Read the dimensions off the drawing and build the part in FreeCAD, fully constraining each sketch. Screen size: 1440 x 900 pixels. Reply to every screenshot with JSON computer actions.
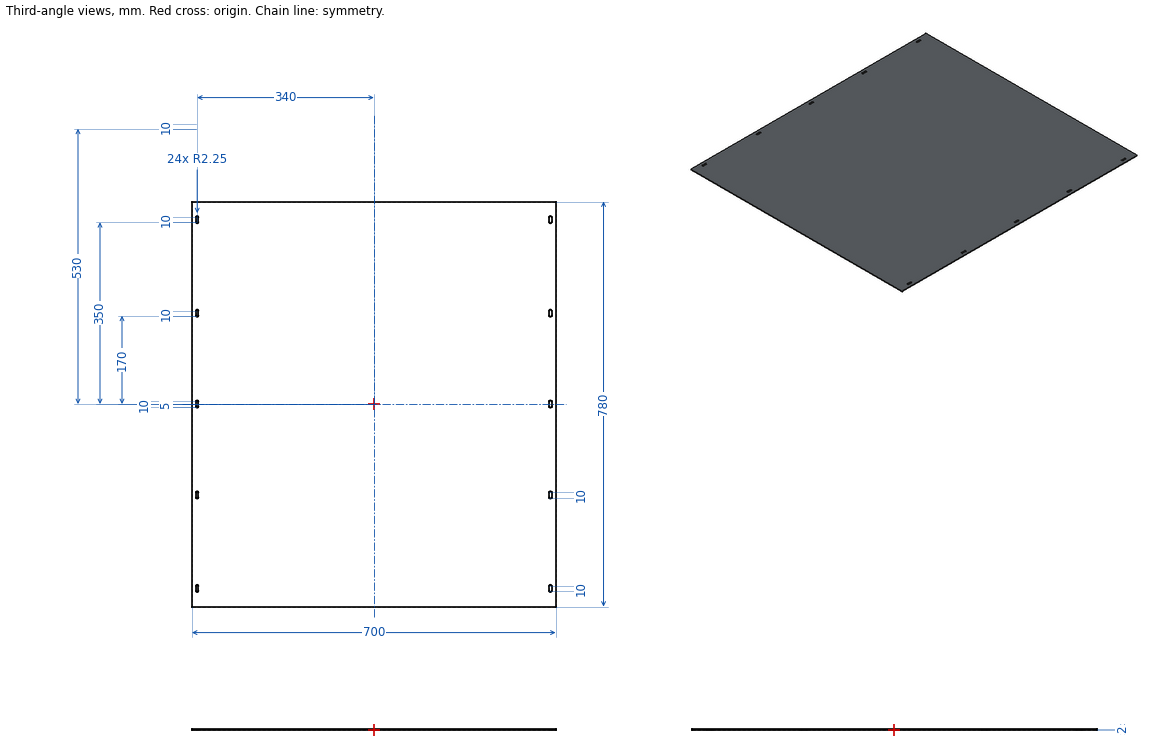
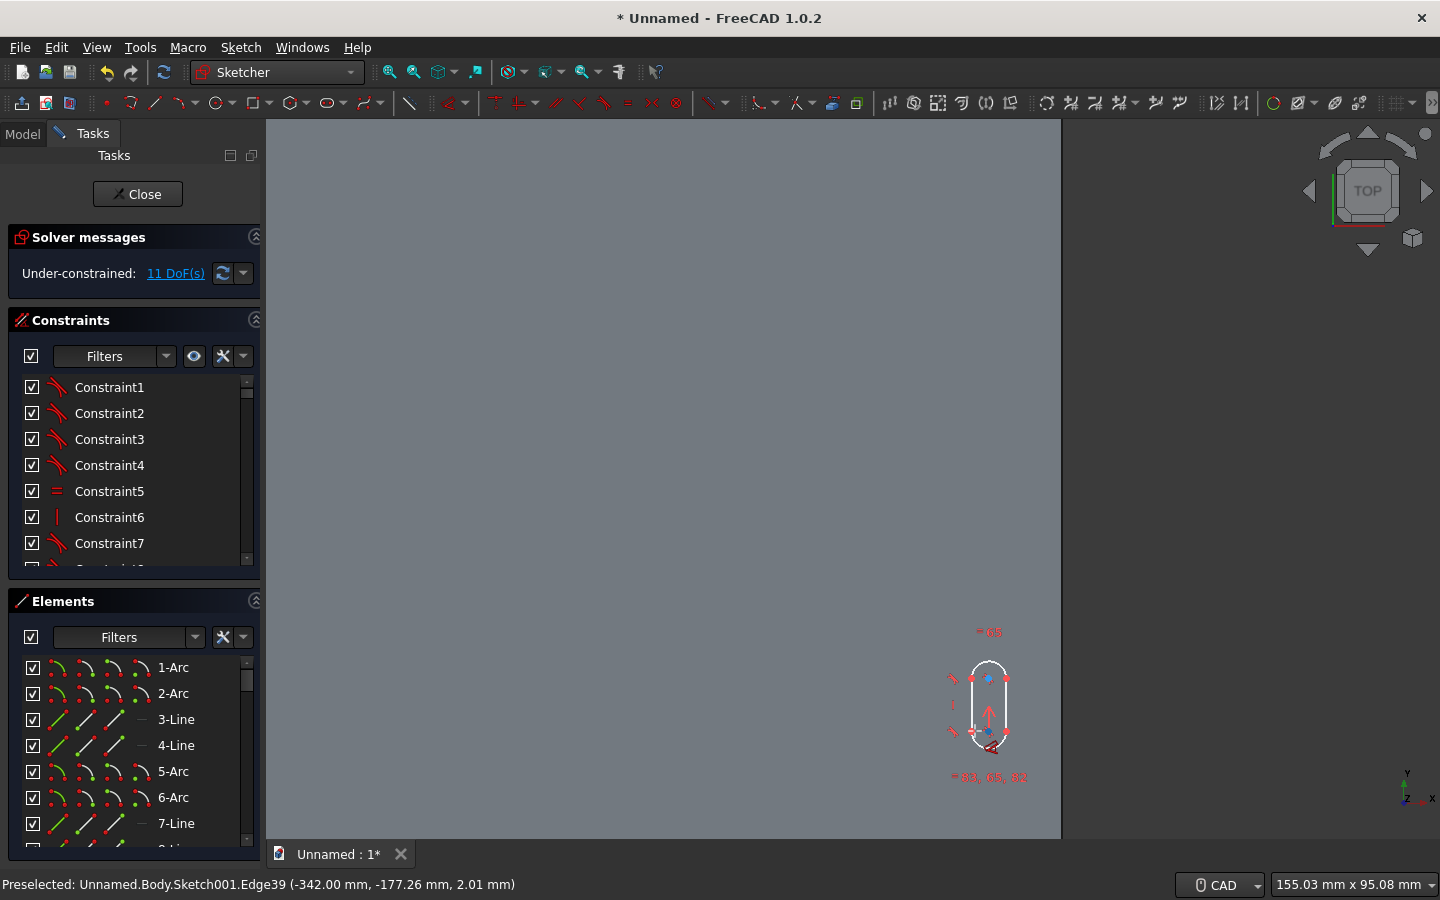
{"action": "left_click", "coordinate": [972, 715]}
{"action": "left_click", "coordinate": [938, 705]}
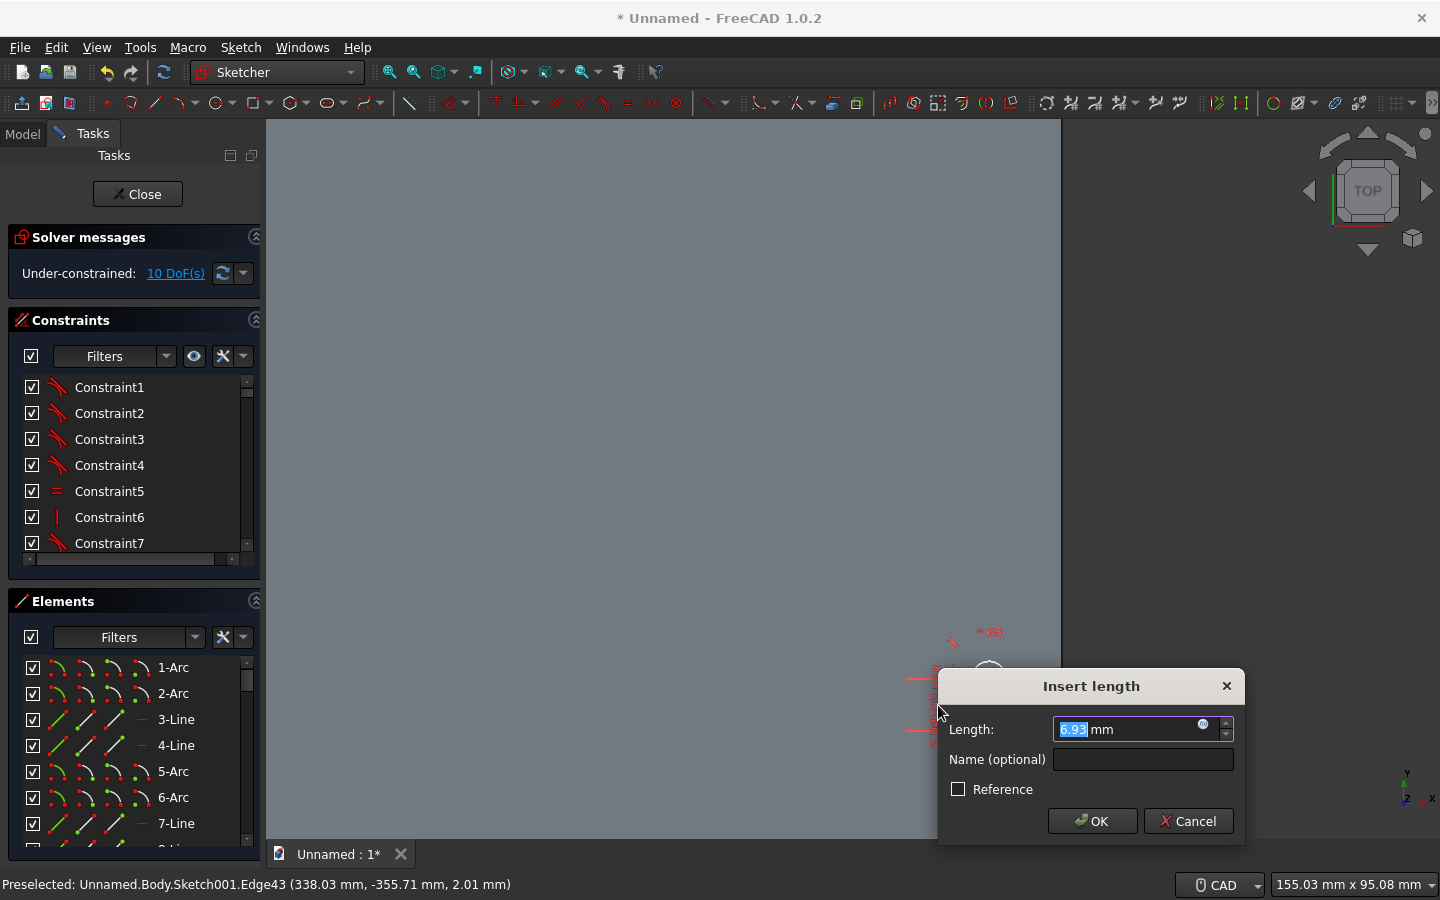
{"action": "type", "text": "10"}
{"action": "key", "text": "Return"}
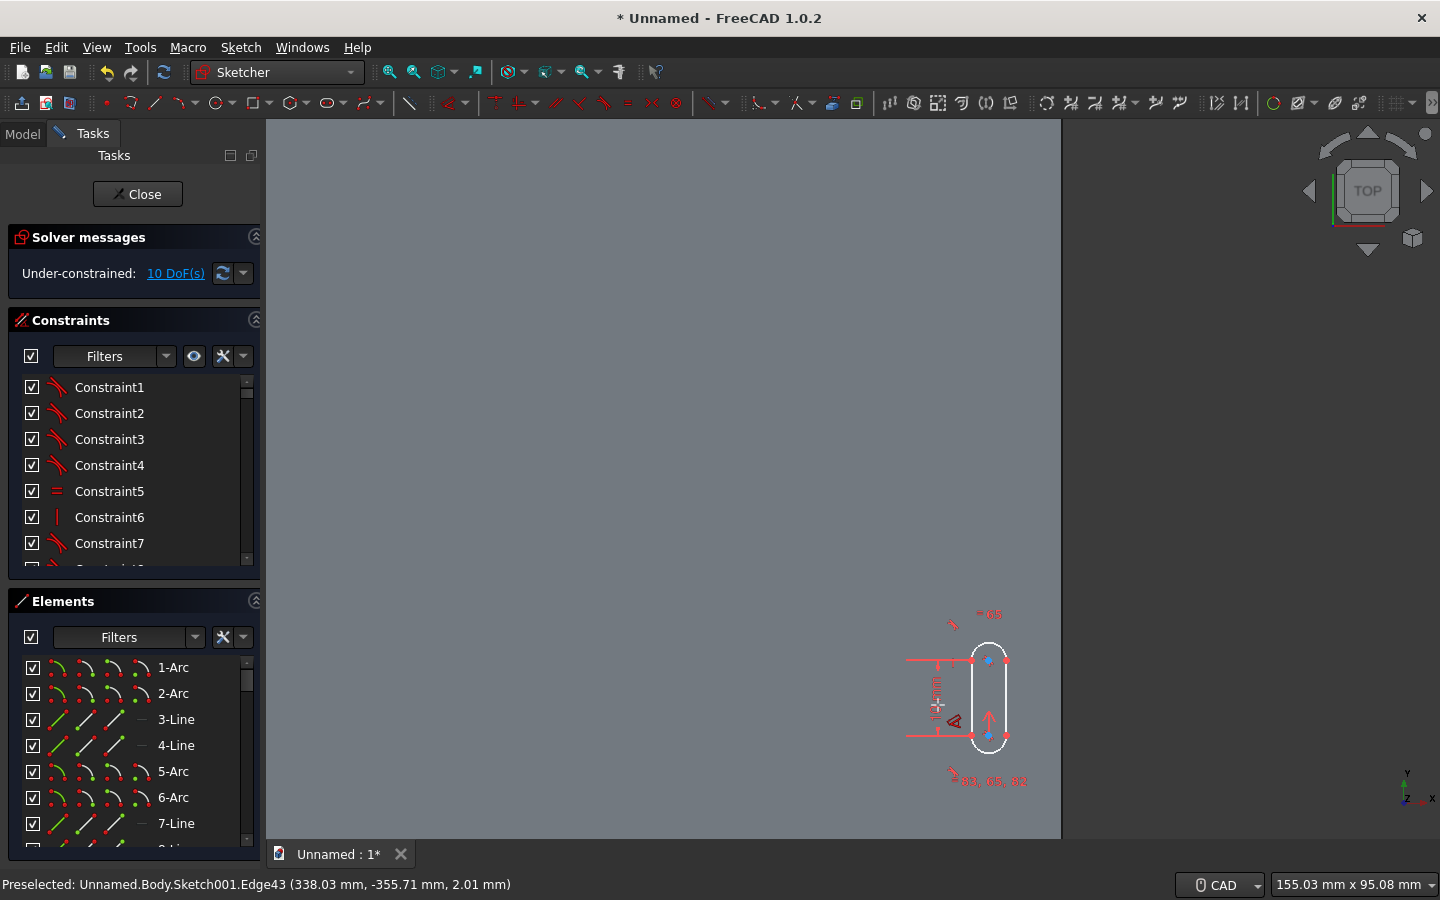
{"action": "scroll", "coordinate": [975, 731], "scroll_direction": "down", "scroll_amount": 13}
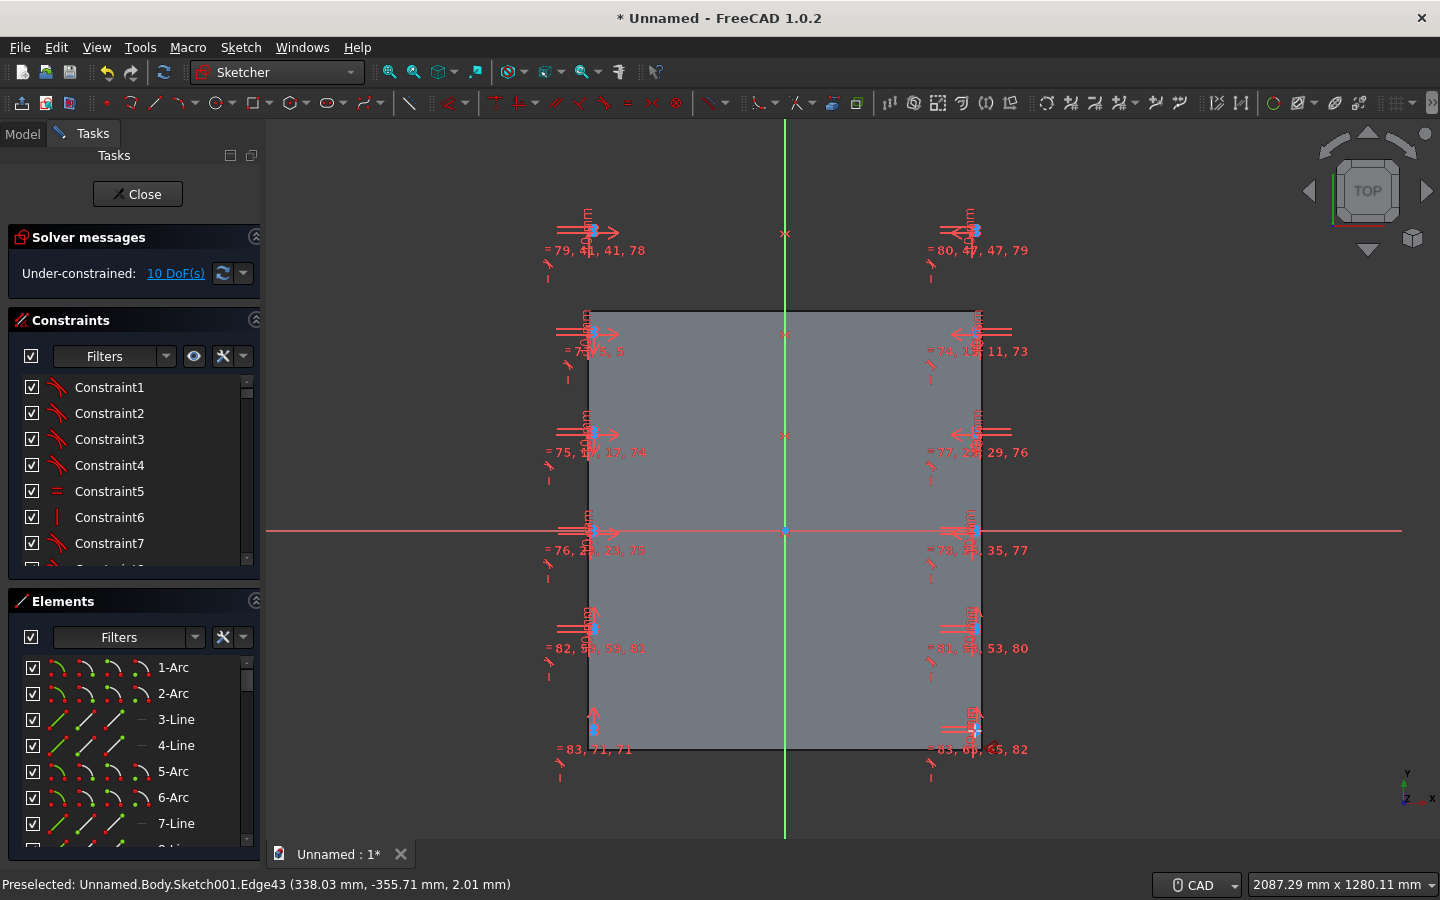
{"action": "scroll", "coordinate": [592, 731], "scroll_direction": "up", "scroll_amount": 12}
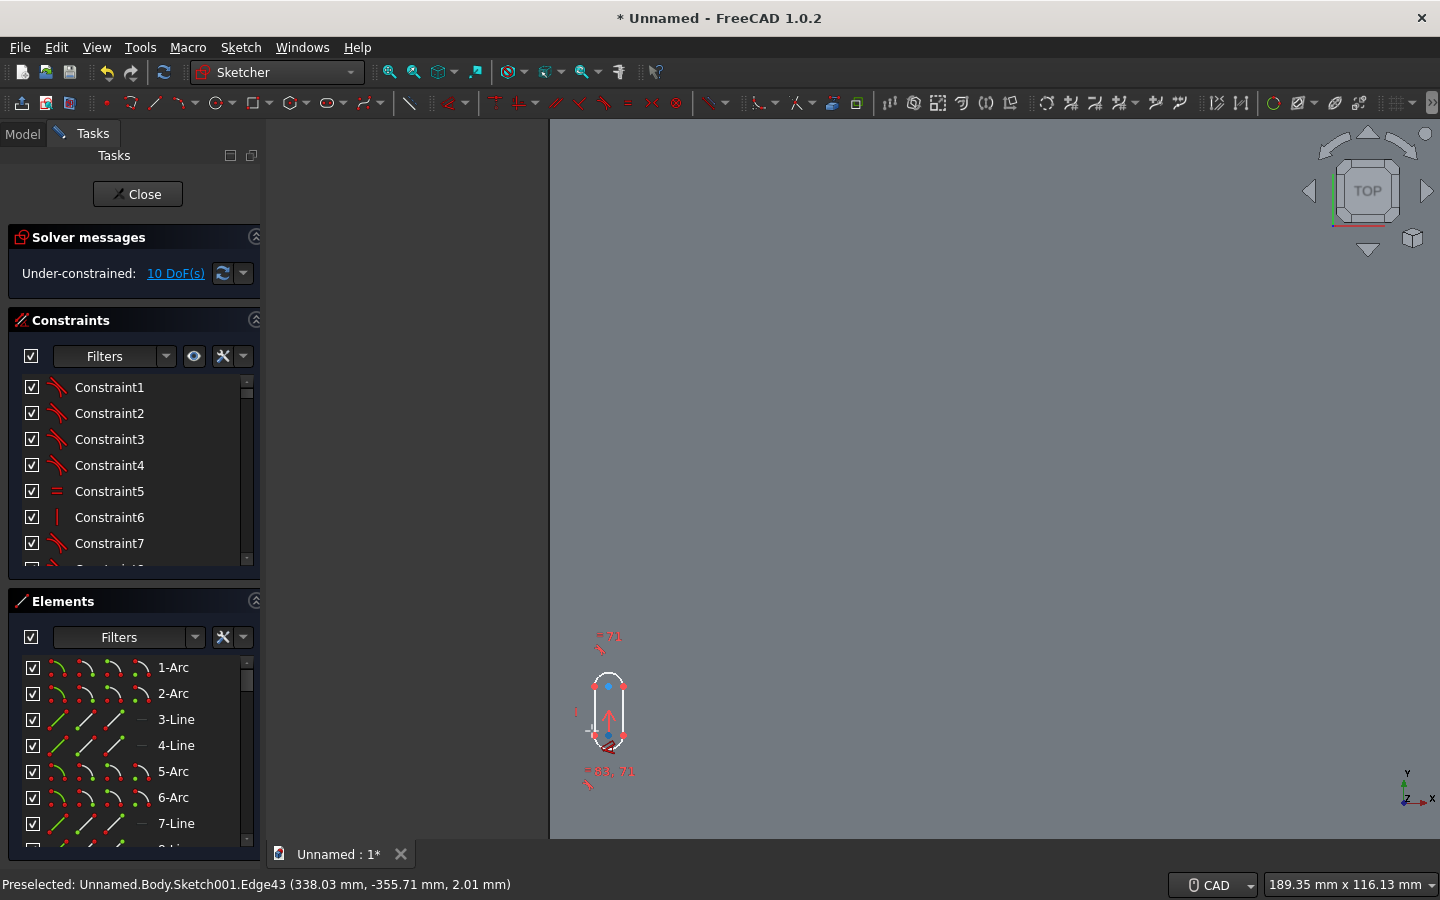
{"action": "left_click", "coordinate": [595, 721]}
{"action": "left_click", "coordinate": [561, 711]}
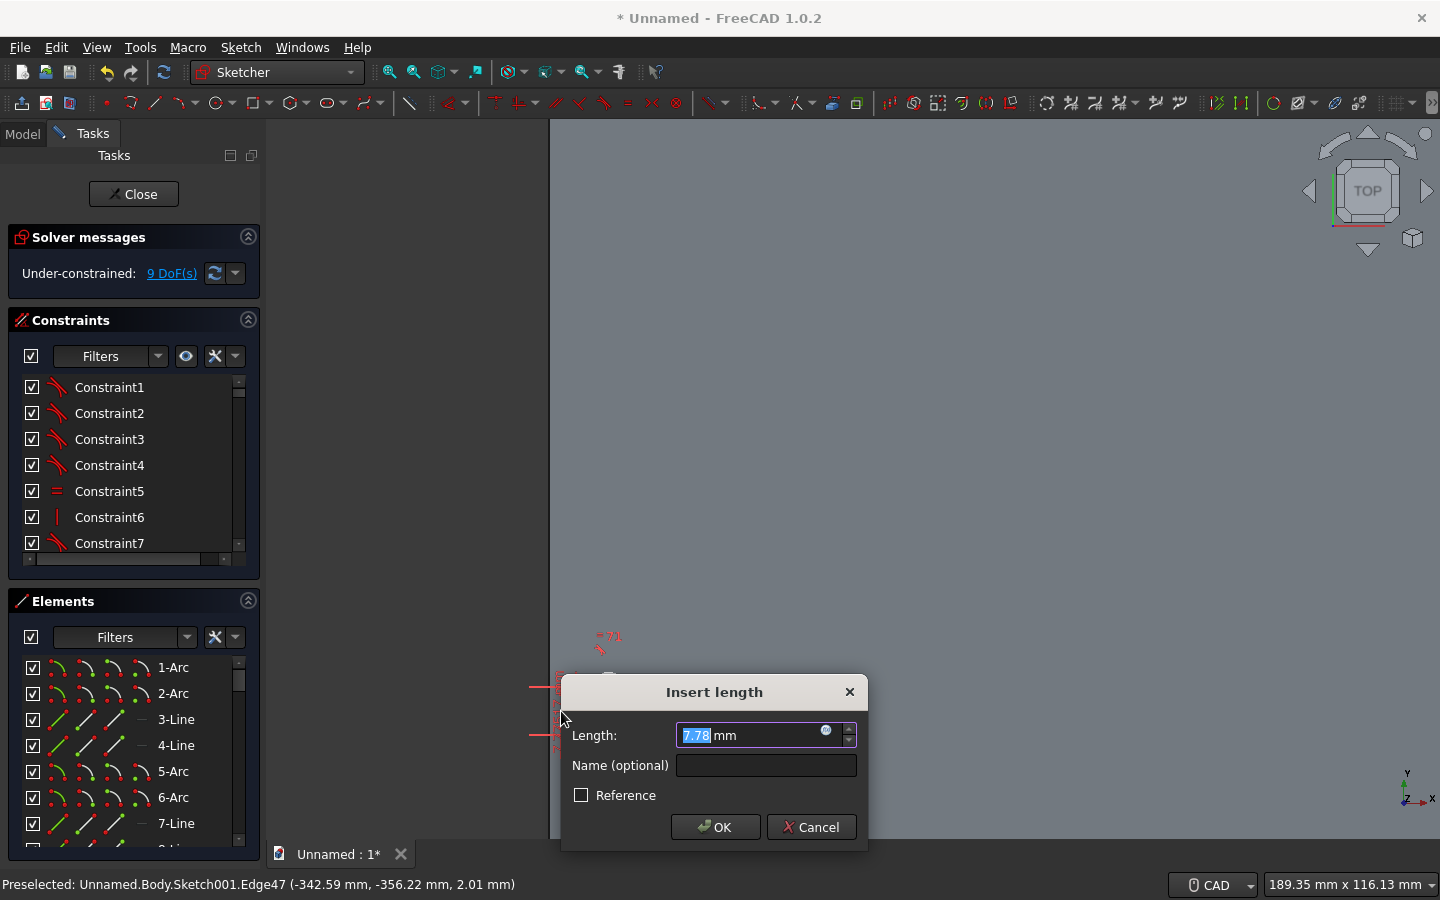
{"action": "type", "text": "10"}
{"action": "key", "text": "Return"}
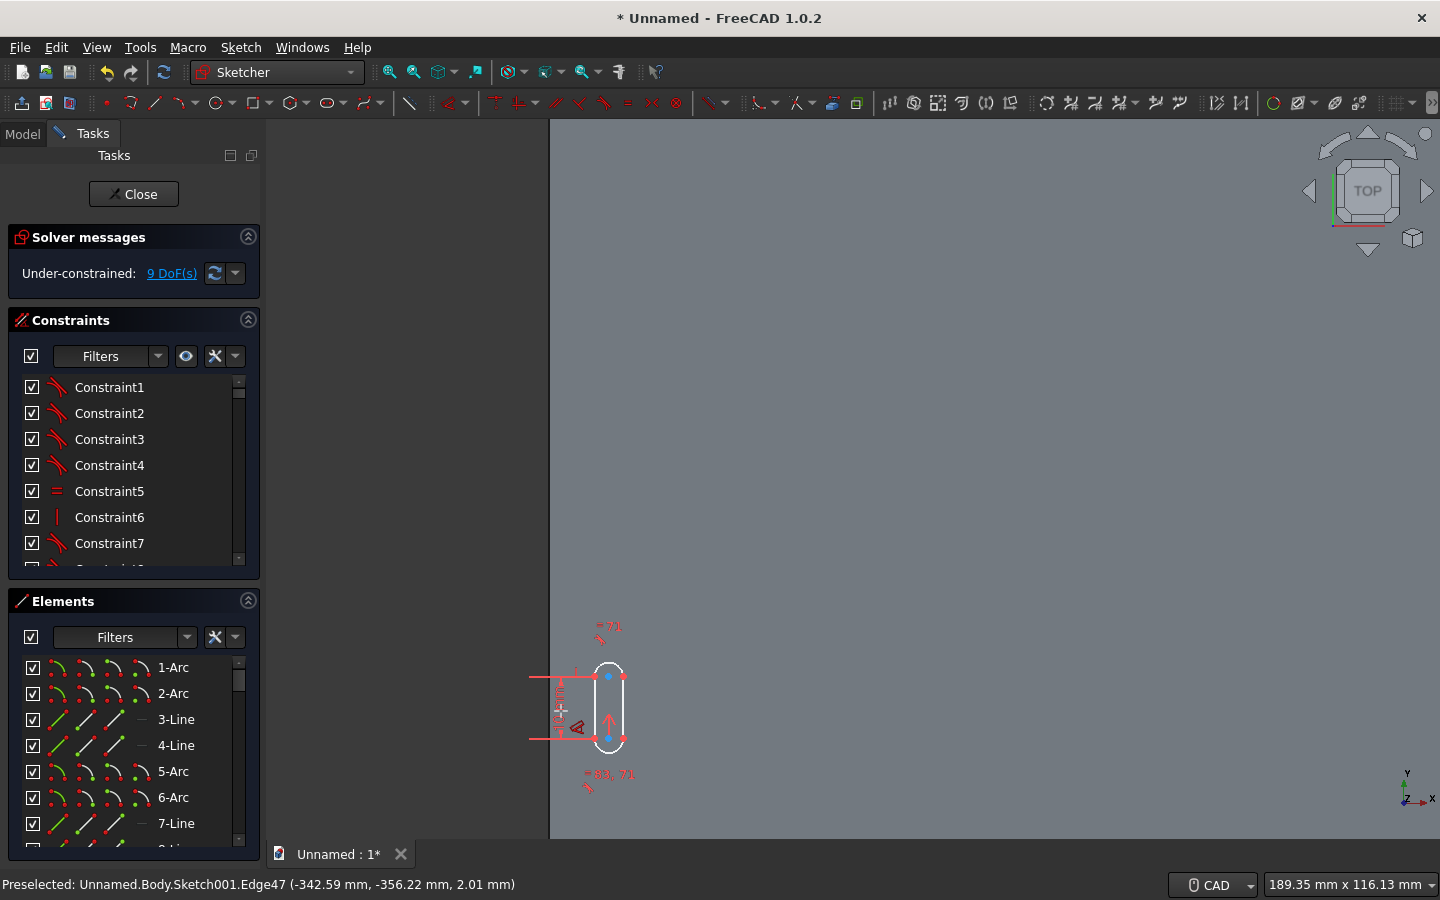
{"action": "scroll", "coordinate": [592, 731], "scroll_direction": "down", "scroll_amount": 12}